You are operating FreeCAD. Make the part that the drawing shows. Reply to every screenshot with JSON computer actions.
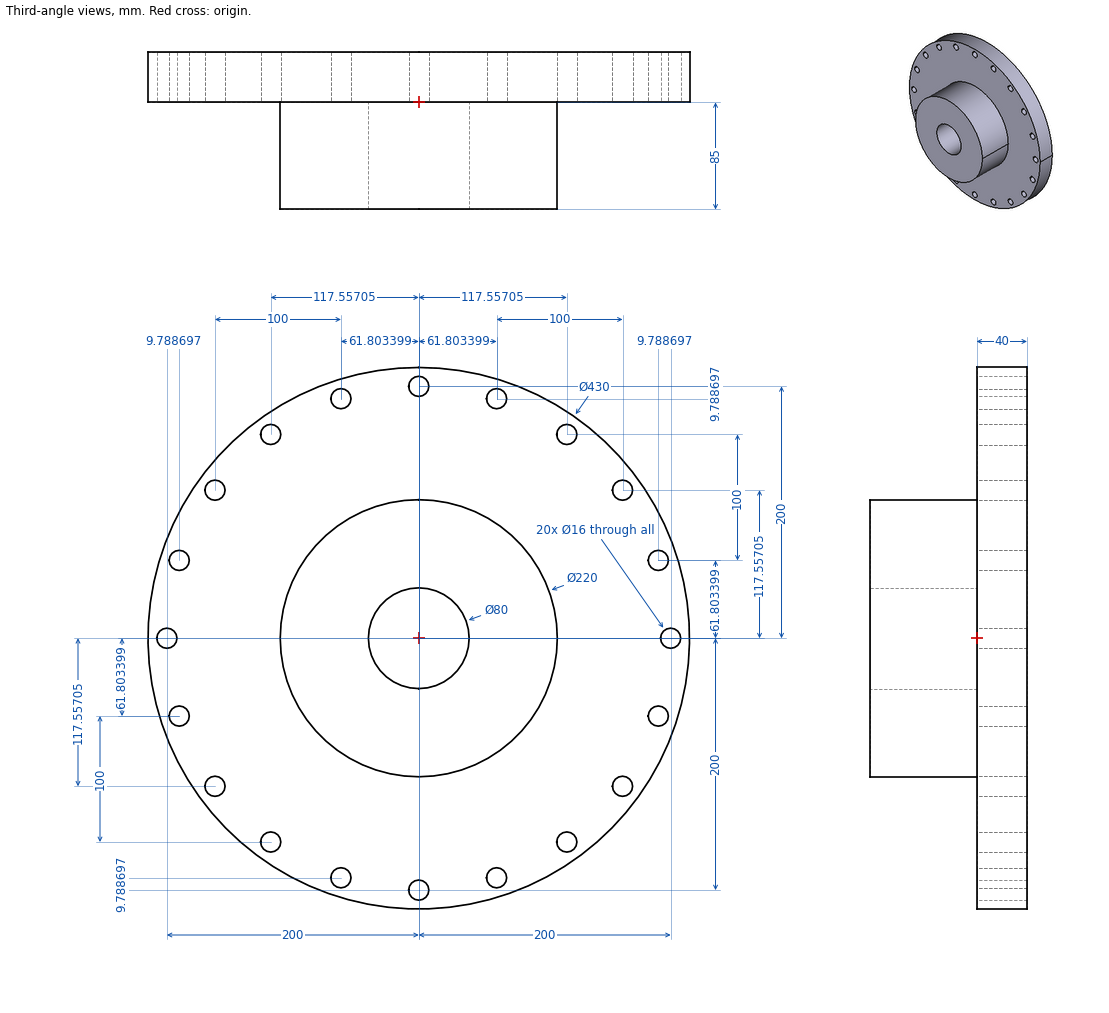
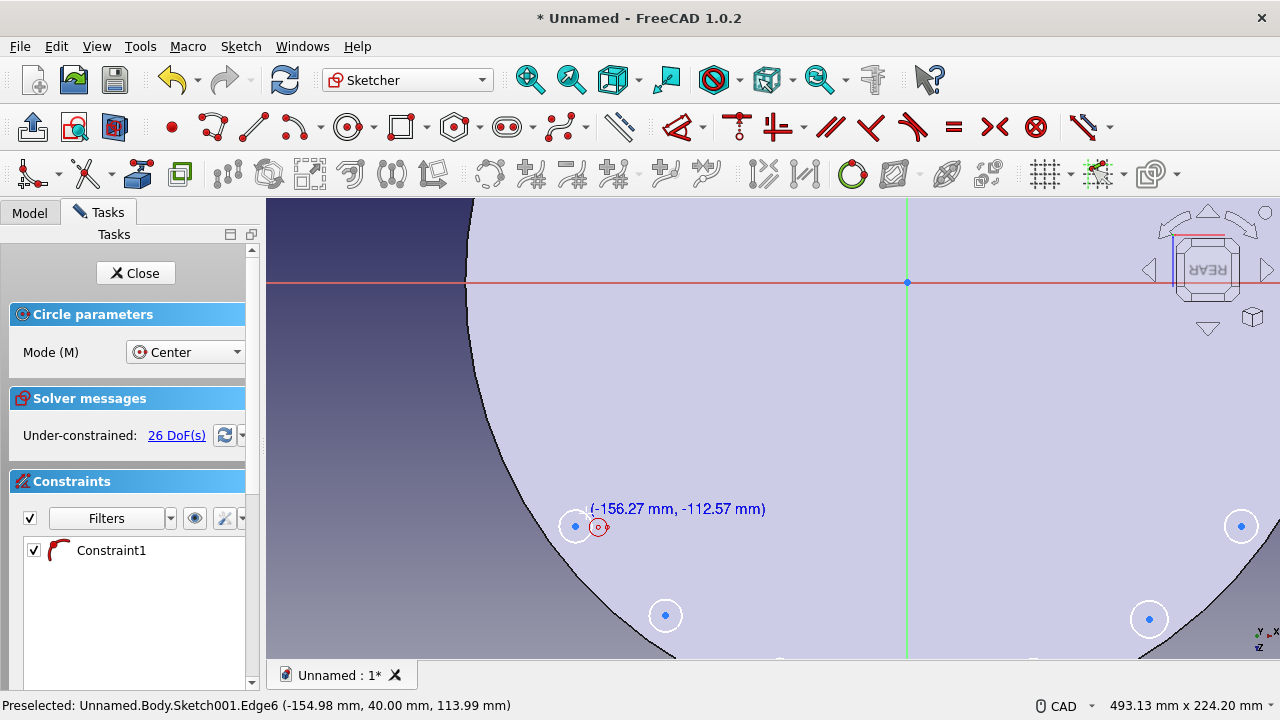
{"action": "scroll", "coordinate": [516, 410], "scroll_direction": "up", "scroll_amount": 2}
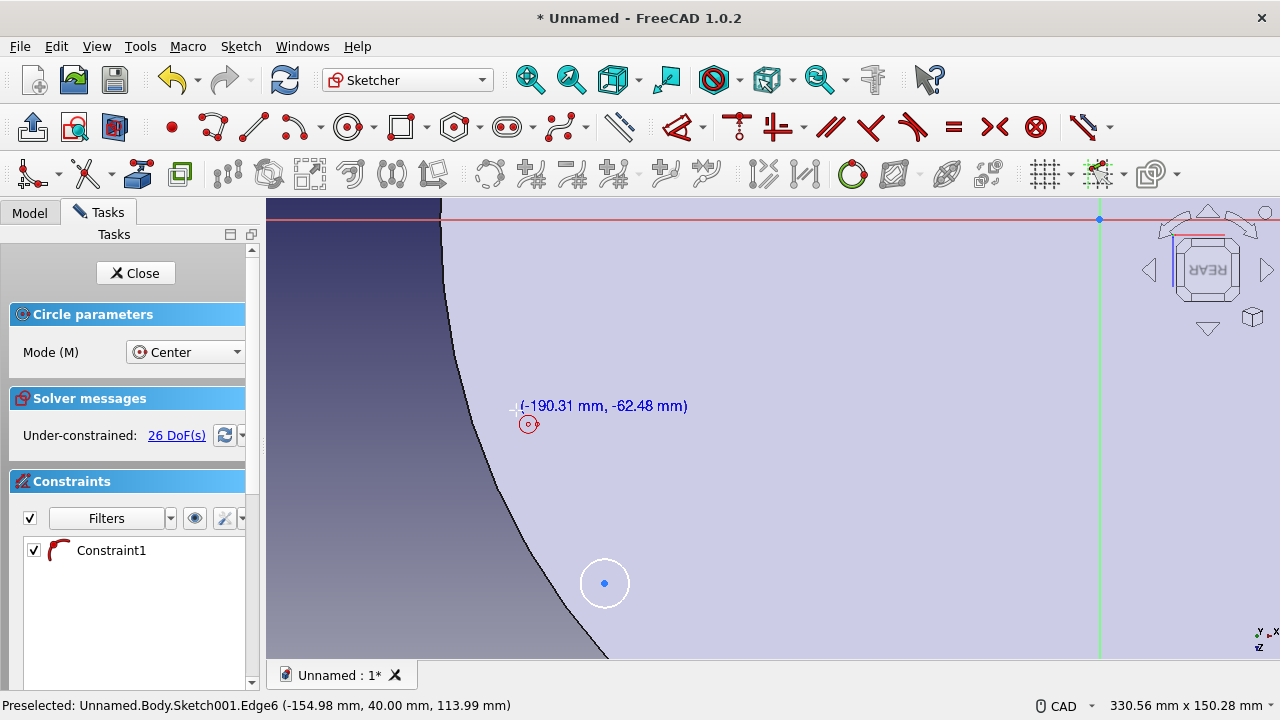
{"action": "scroll", "coordinate": [575, 497], "scroll_direction": "down", "scroll_amount": 7}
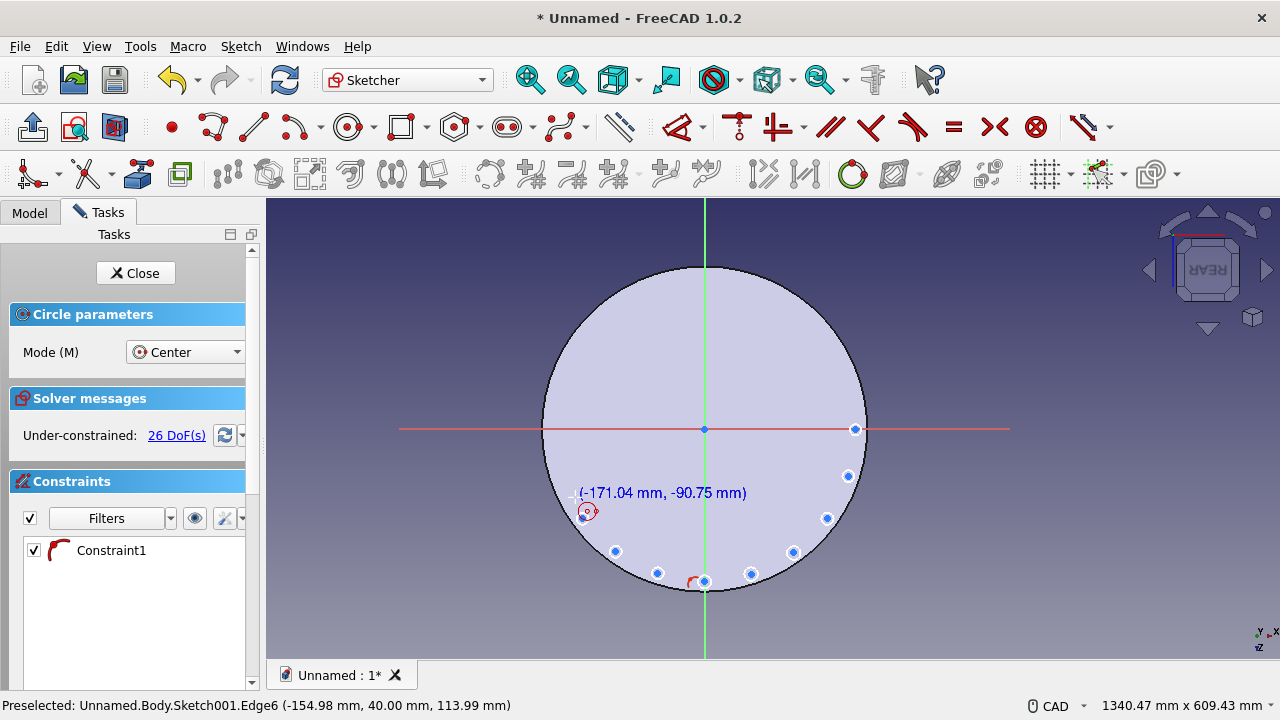
{"action": "left_click", "coordinate": [561, 476]}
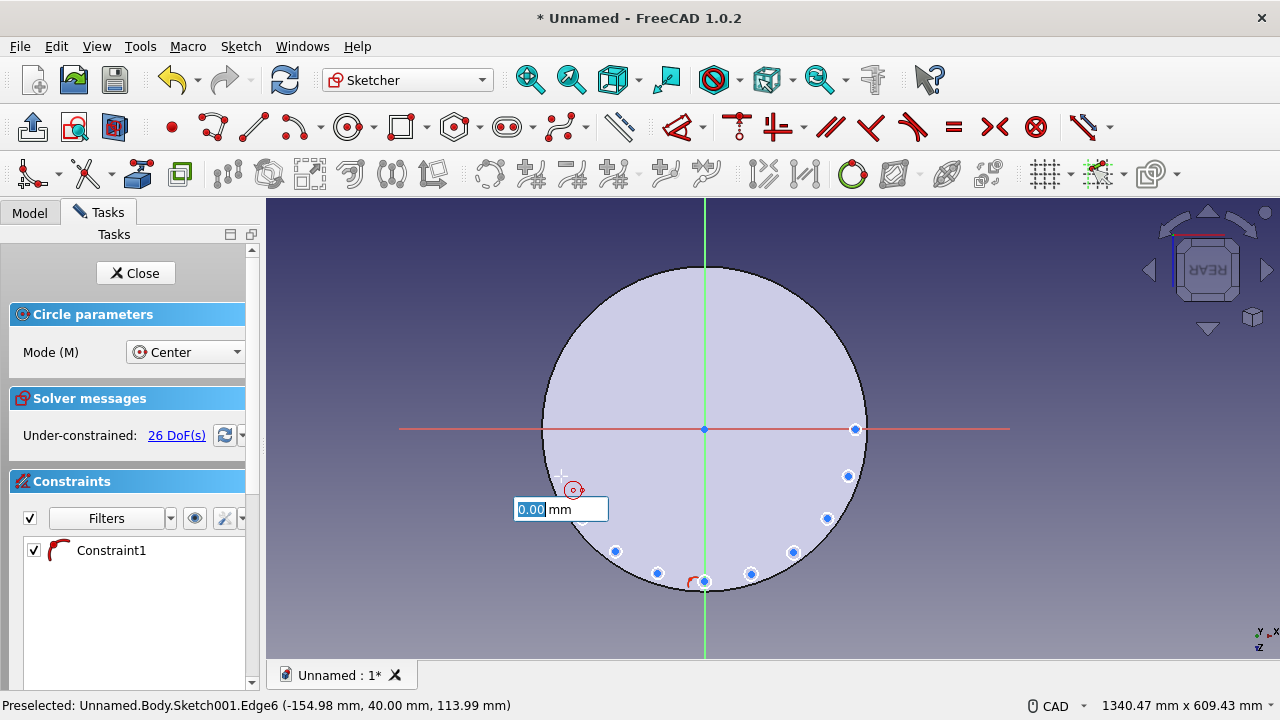
{"action": "scroll", "coordinate": [565, 472], "scroll_direction": "up", "scroll_amount": 5}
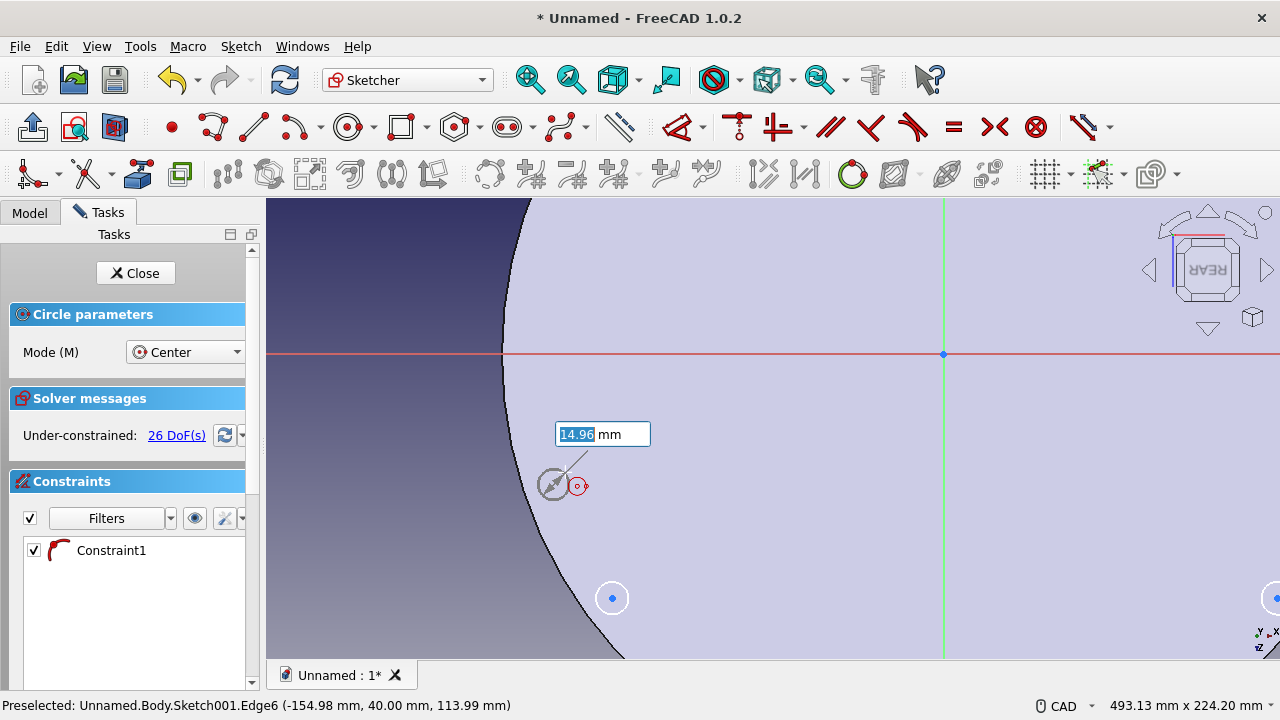
{"action": "left_click", "coordinate": [565, 470]}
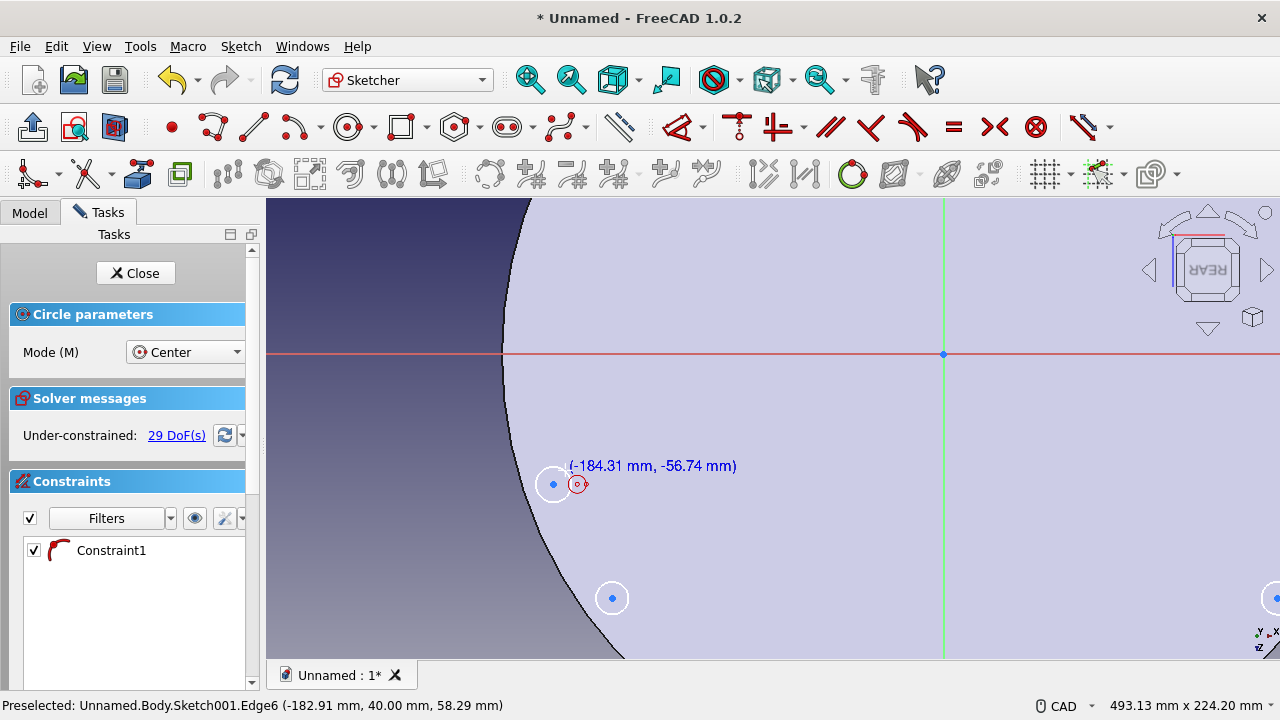
{"action": "scroll", "coordinate": [533, 354], "scroll_direction": "up", "scroll_amount": 2}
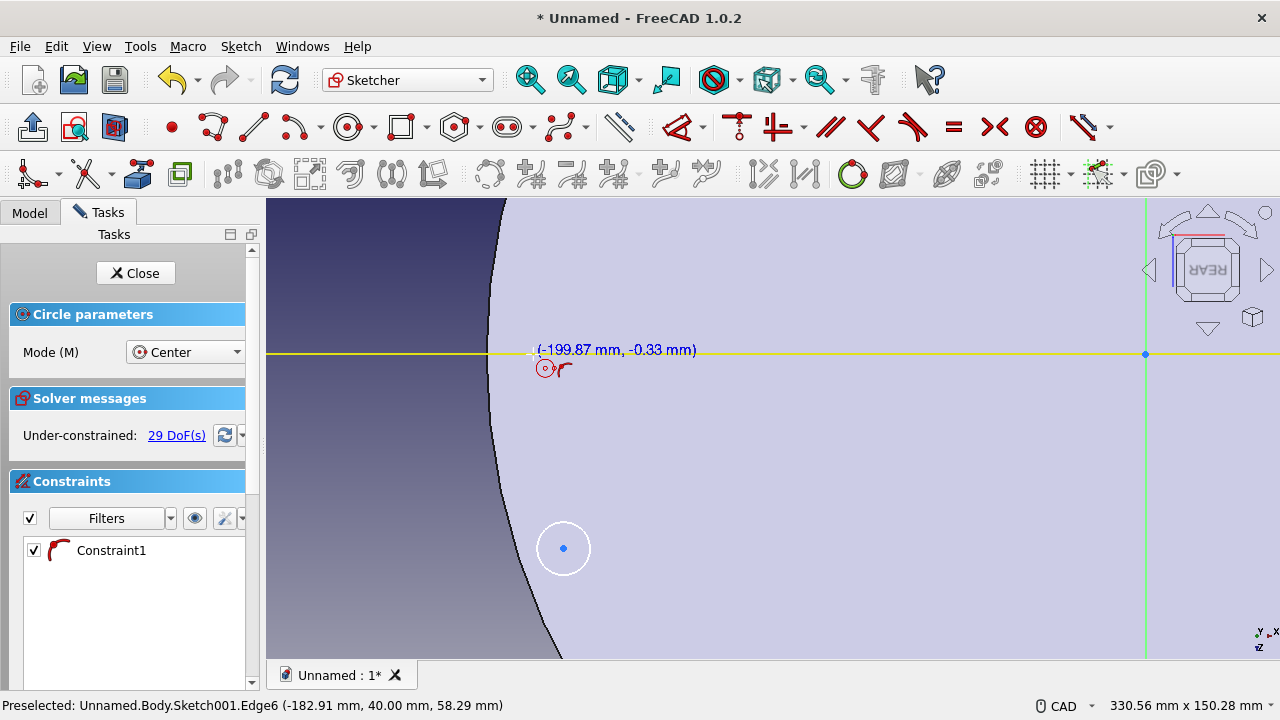
{"action": "scroll", "coordinate": [560, 453], "scroll_direction": "down", "scroll_amount": 7}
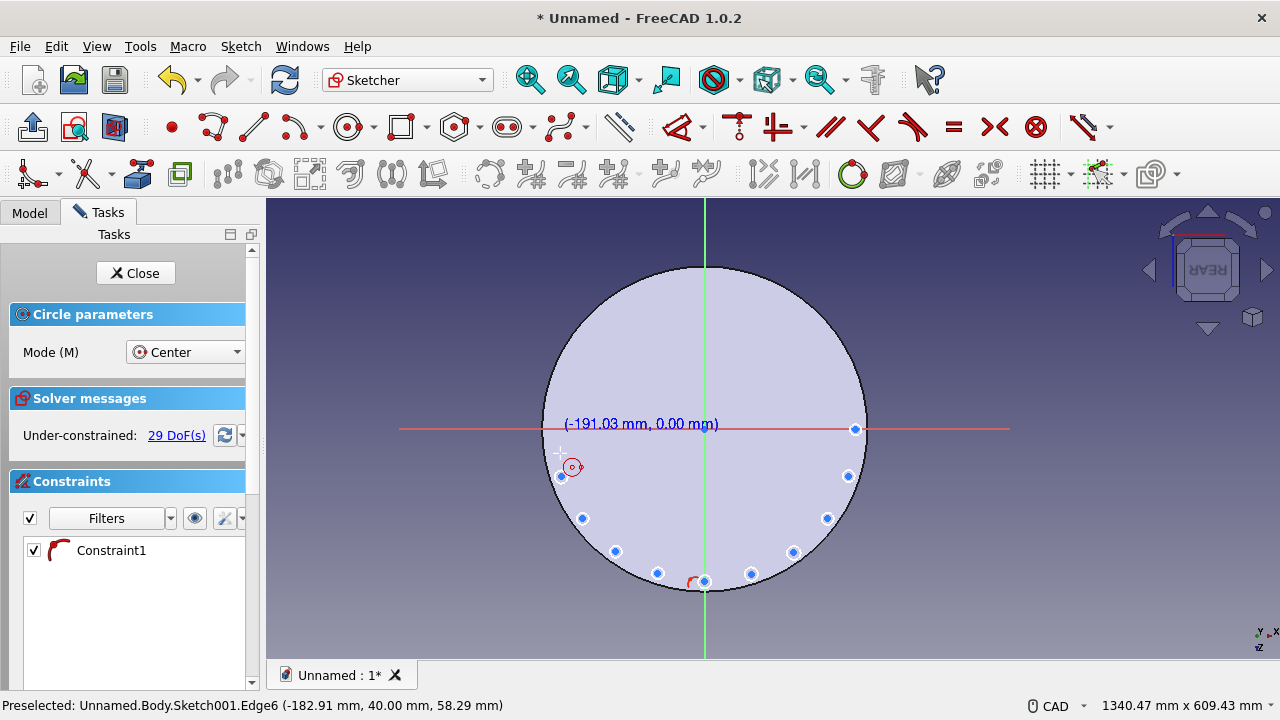
{"action": "left_click", "coordinate": [553, 429]}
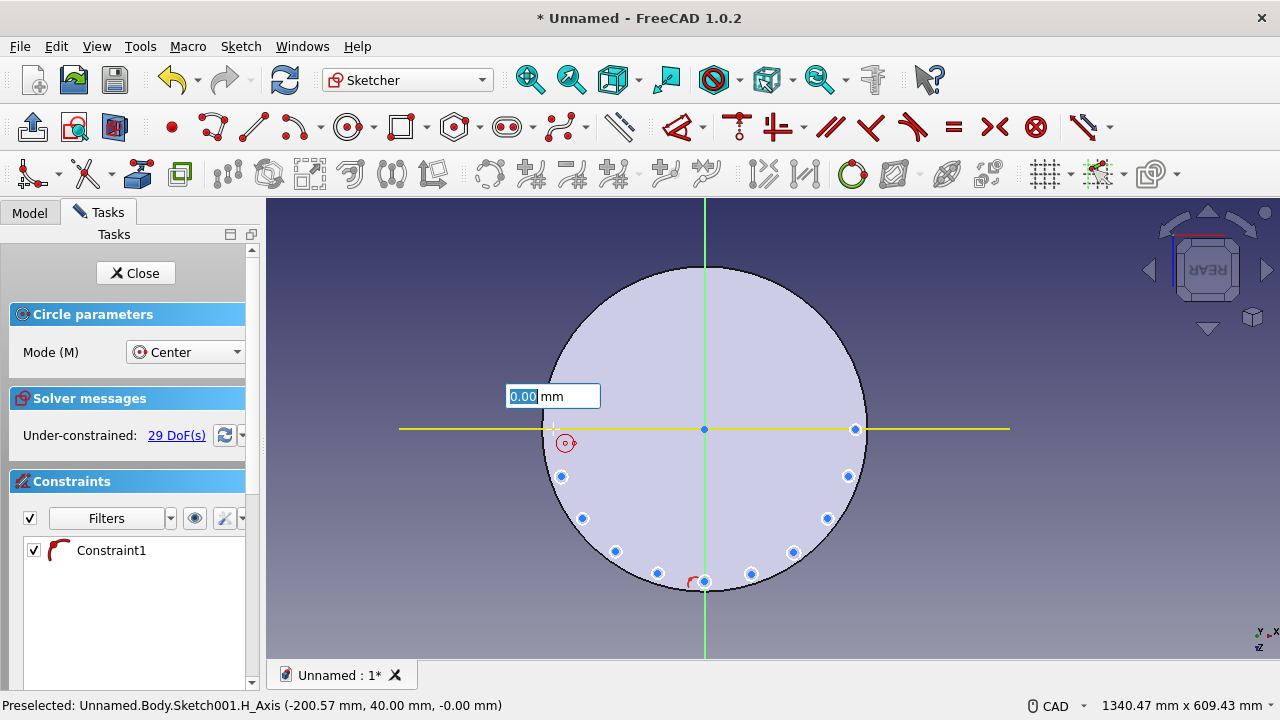
{"action": "scroll", "coordinate": [551, 435], "scroll_direction": "up", "scroll_amount": 6}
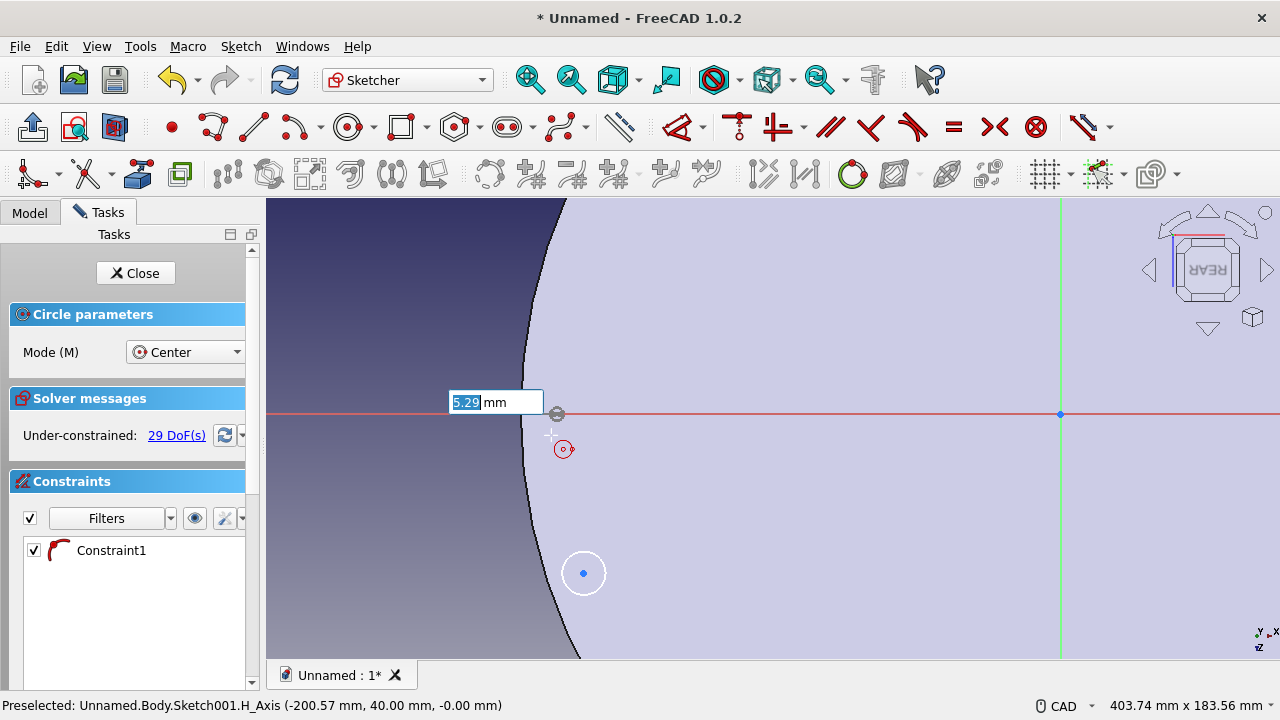
{"action": "left_click", "coordinate": [552, 433]}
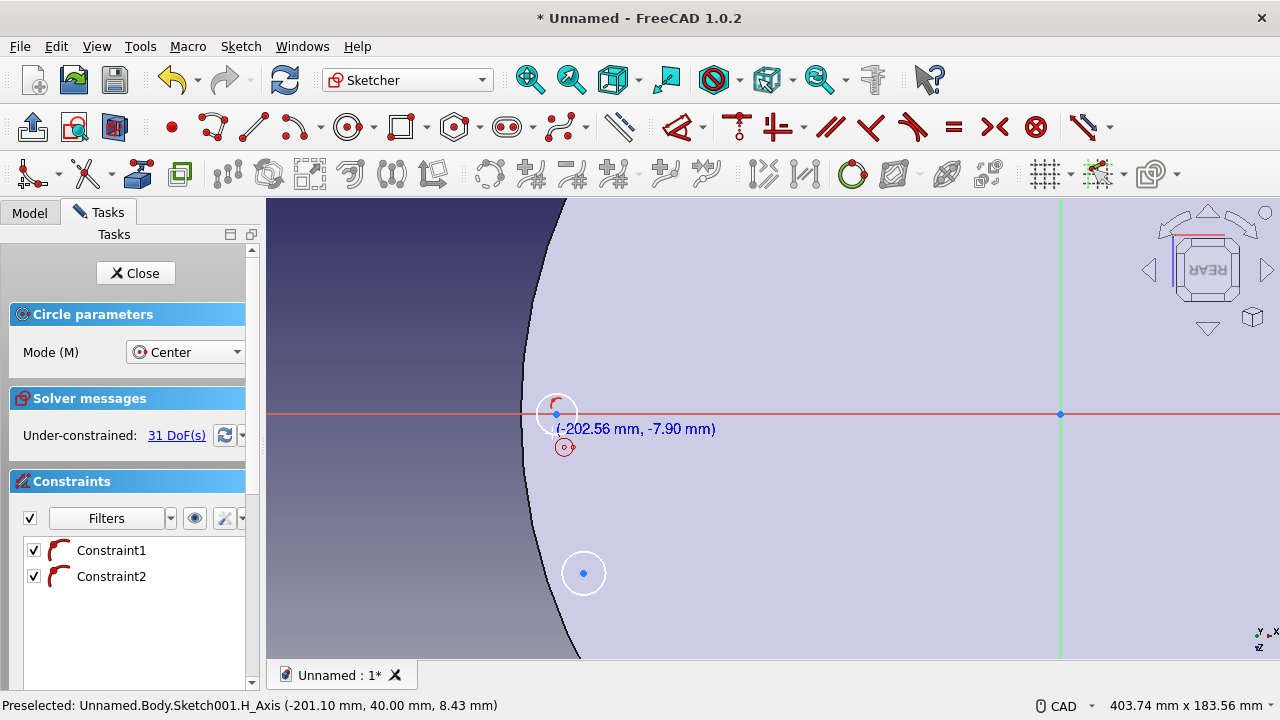
{"action": "left_click", "coordinate": [583, 259]}
{"action": "left_click", "coordinate": [597, 245]}